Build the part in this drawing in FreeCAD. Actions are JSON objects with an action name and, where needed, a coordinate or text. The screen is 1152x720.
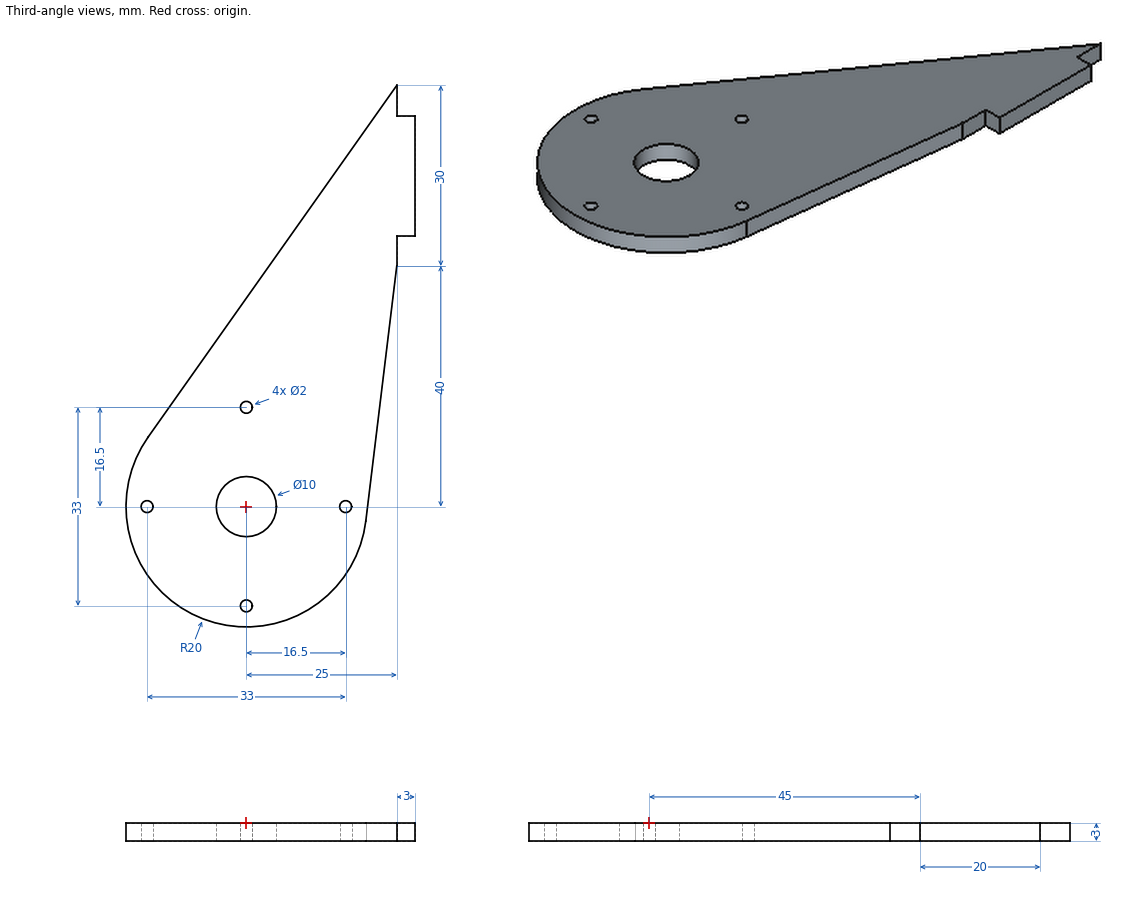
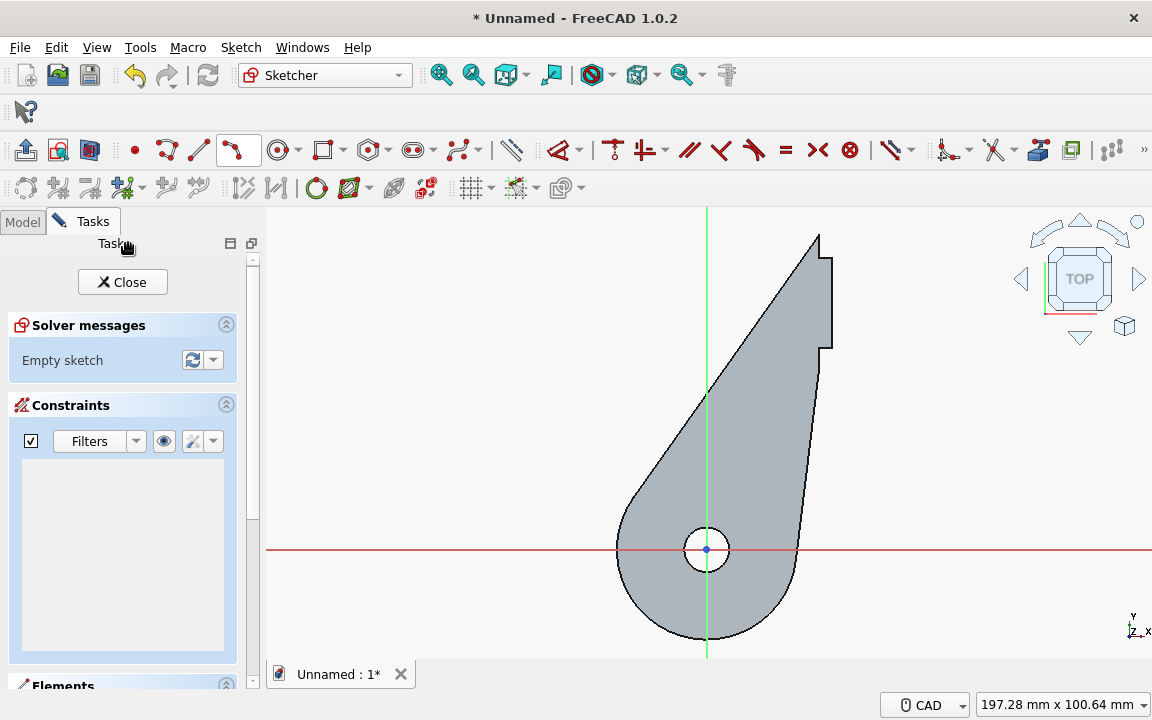
{"action": "scroll", "coordinate": [640, 433], "scroll_direction": "down", "scroll_amount": 5}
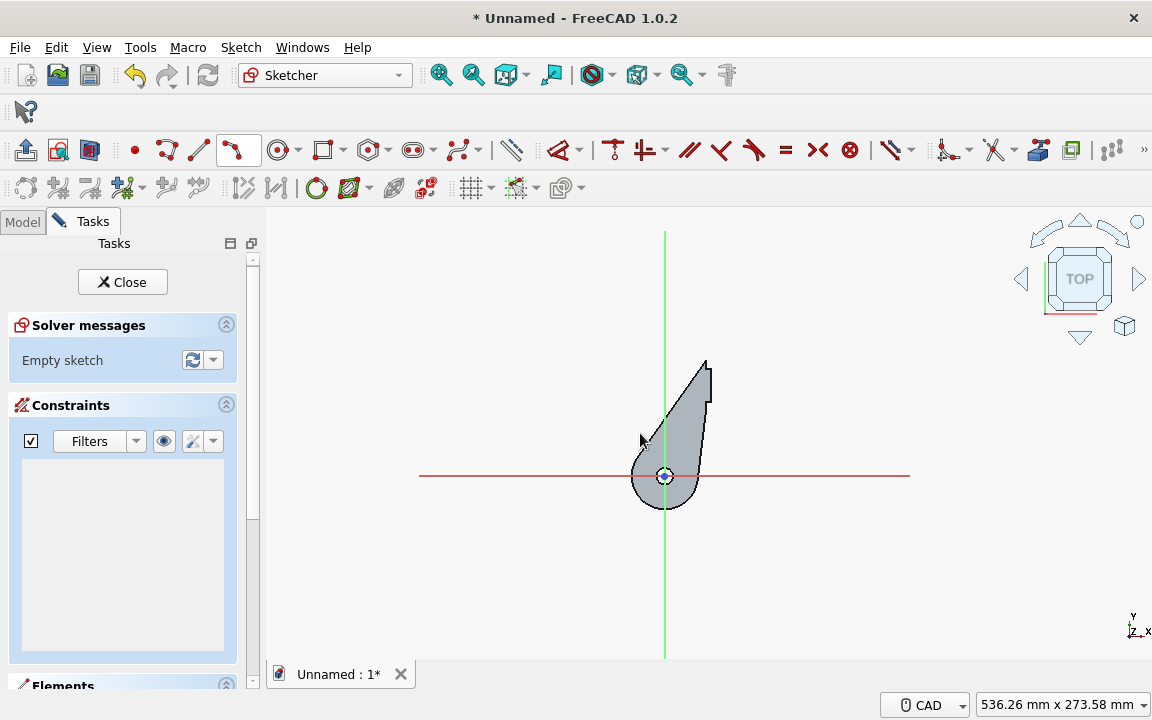
{"action": "scroll", "coordinate": [671, 487], "scroll_direction": "up", "scroll_amount": 8}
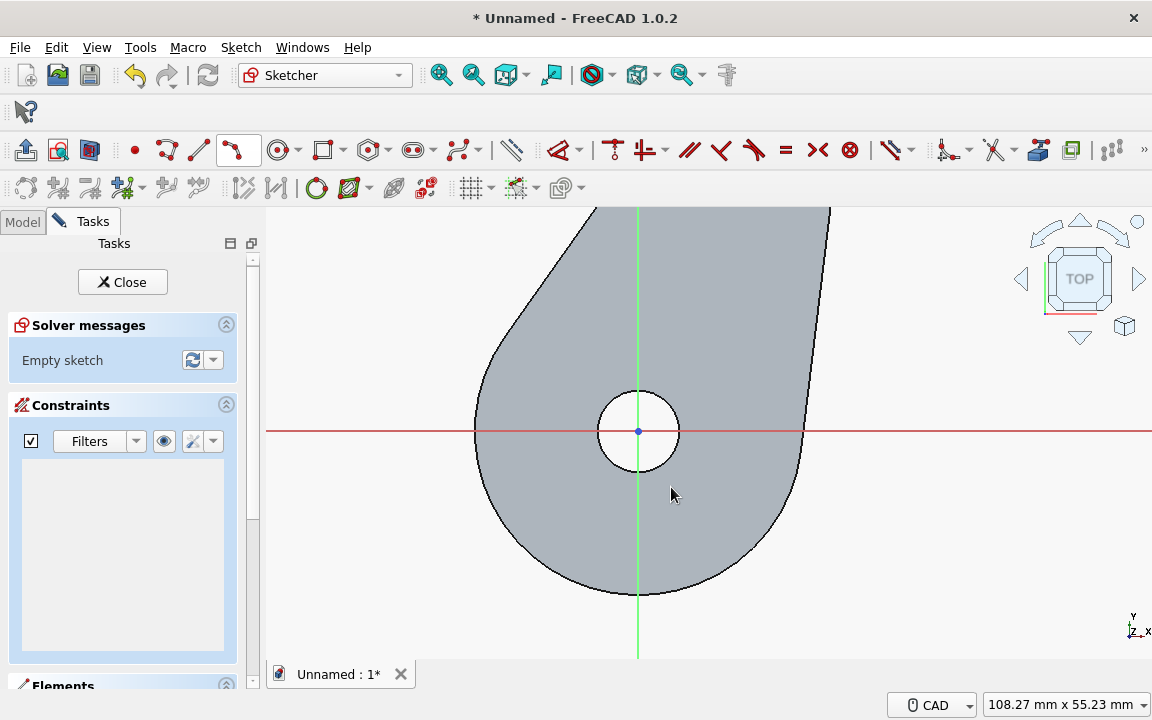
{"action": "left_click", "coordinate": [278, 150]}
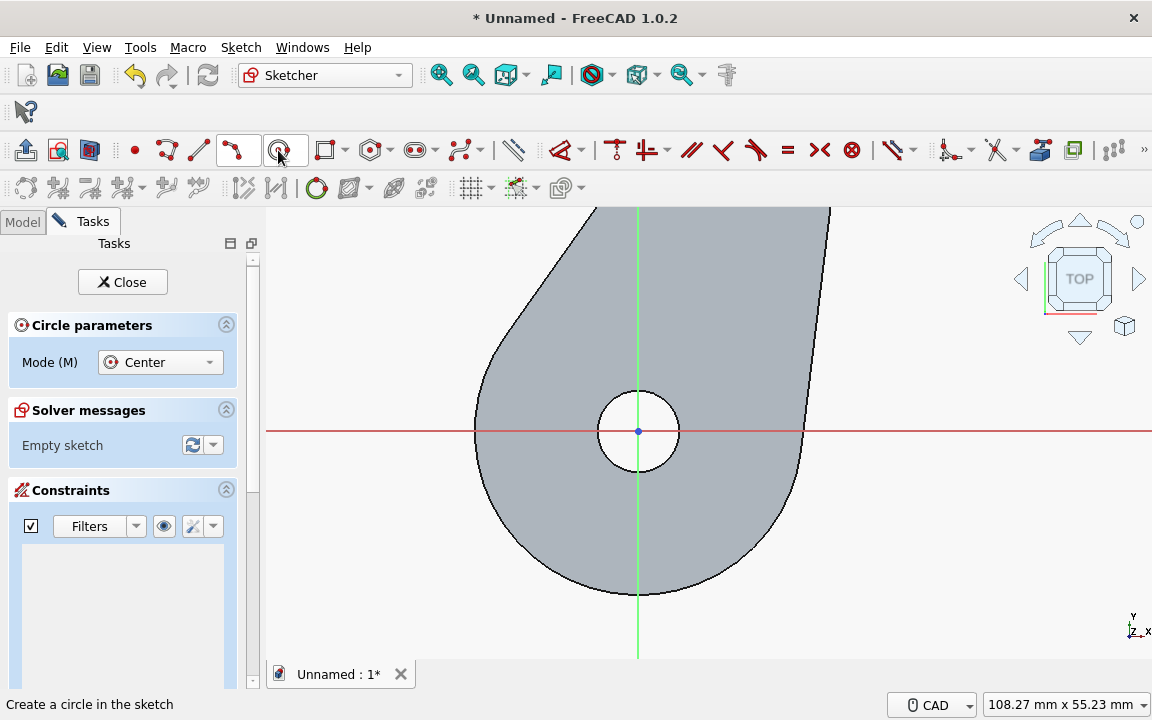
{"action": "scroll", "coordinate": [638, 296], "scroll_direction": "up", "scroll_amount": 6}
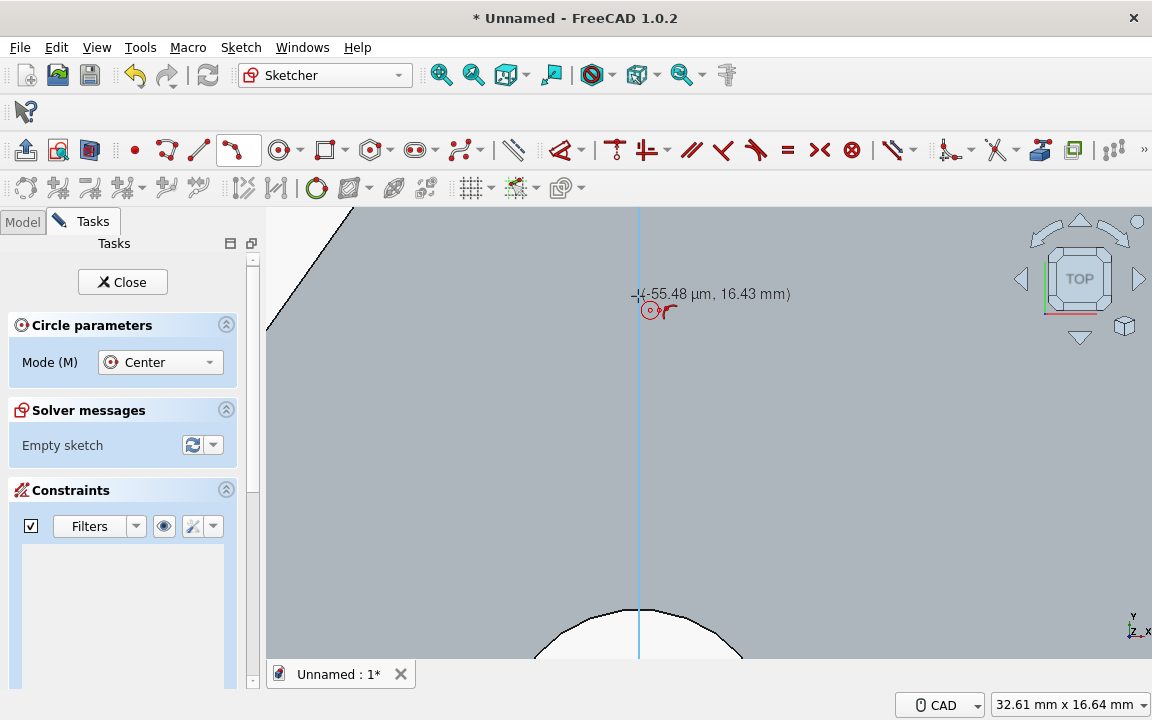
{"action": "left_click", "coordinate": [639, 297]}
{"action": "left_click", "coordinate": [658, 278]}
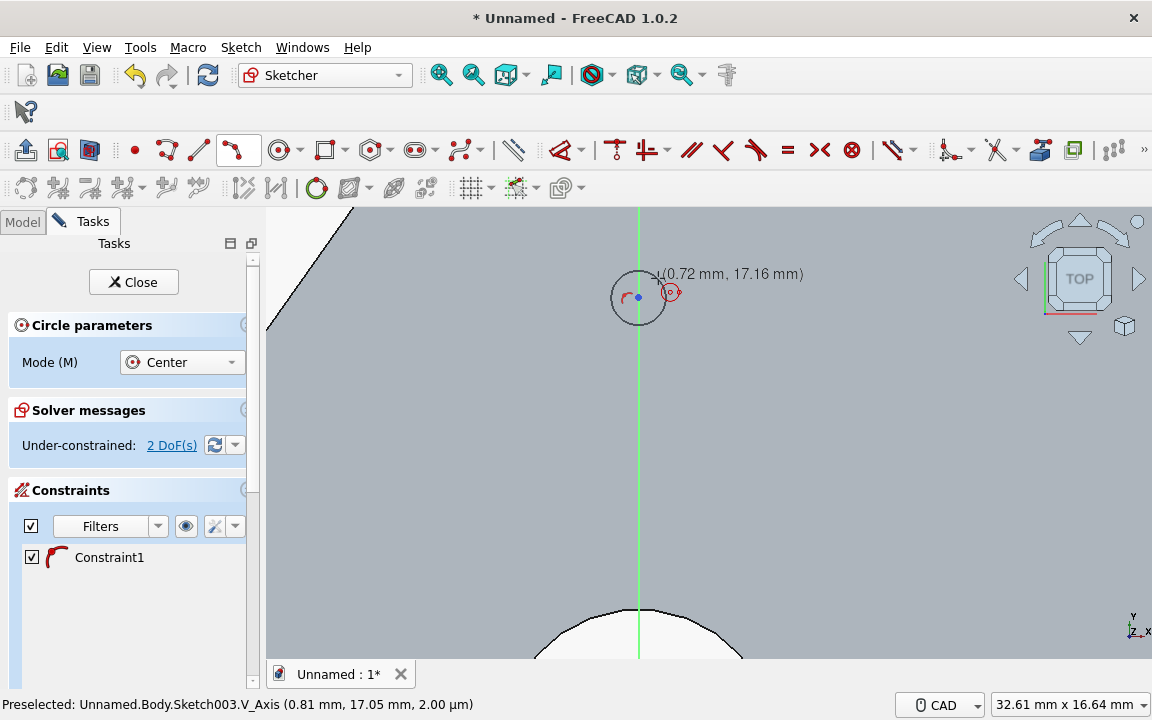
{"action": "scroll", "coordinate": [641, 298], "scroll_direction": "down", "scroll_amount": 6}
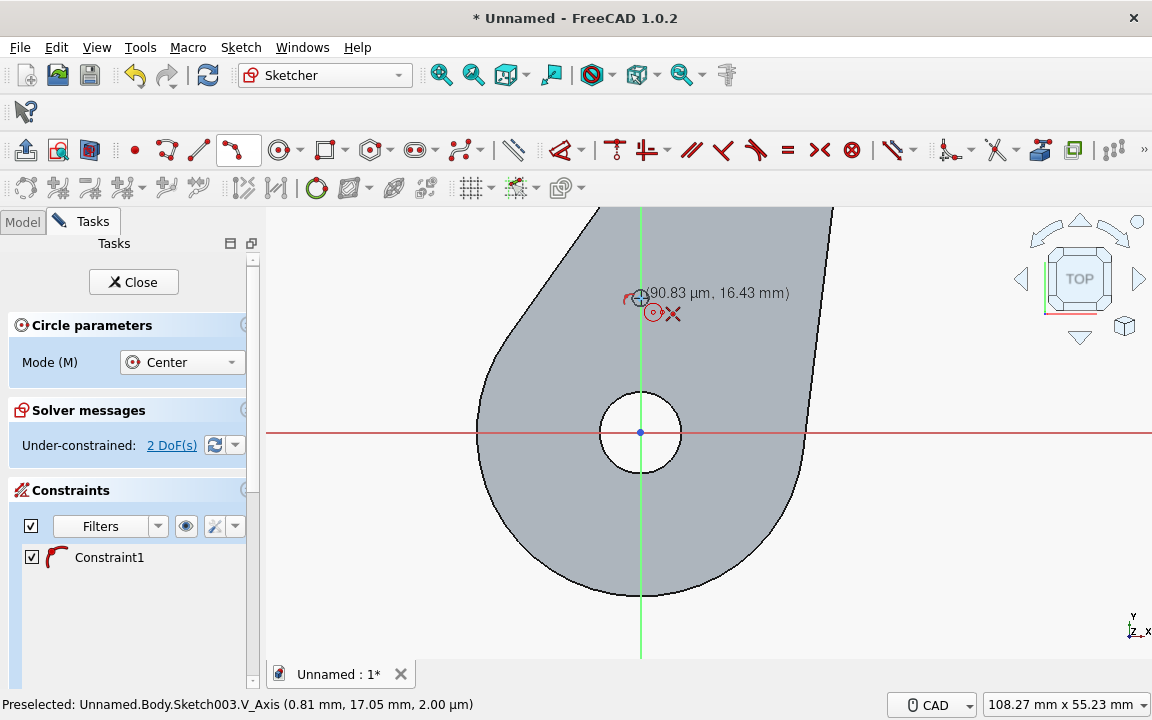
{"action": "scroll", "coordinate": [641, 568], "scroll_direction": "up", "scroll_amount": 6}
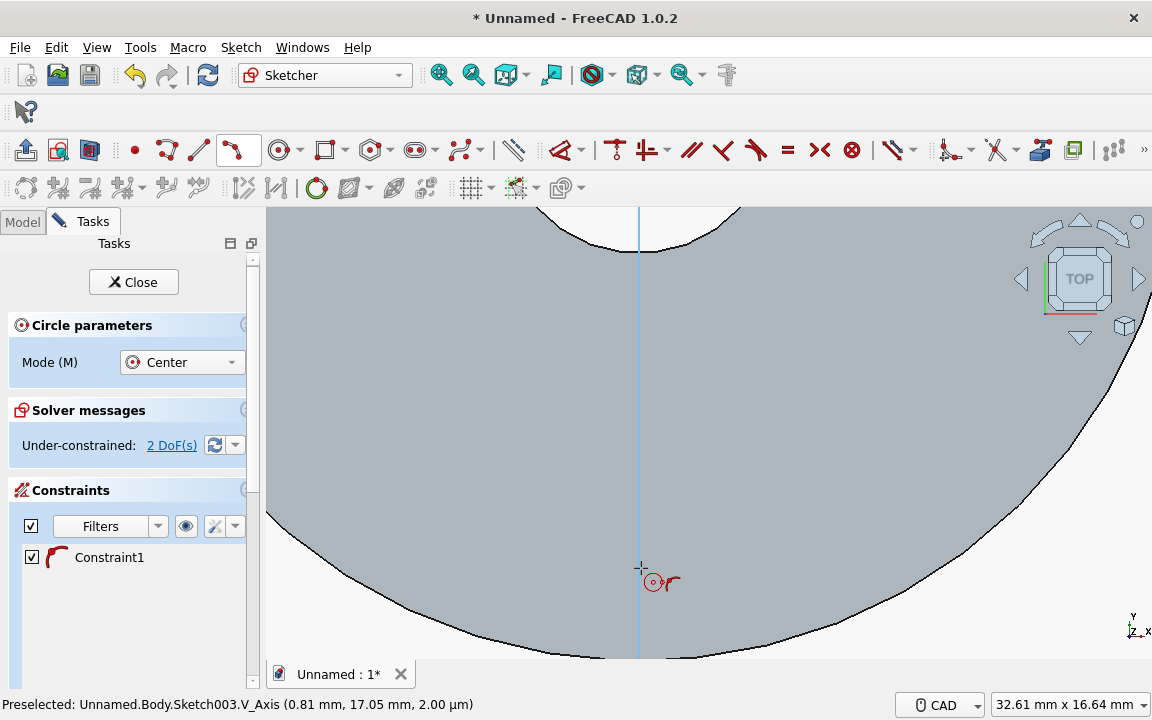
{"action": "left_click", "coordinate": [639, 566]}
{"action": "left_click", "coordinate": [658, 547]}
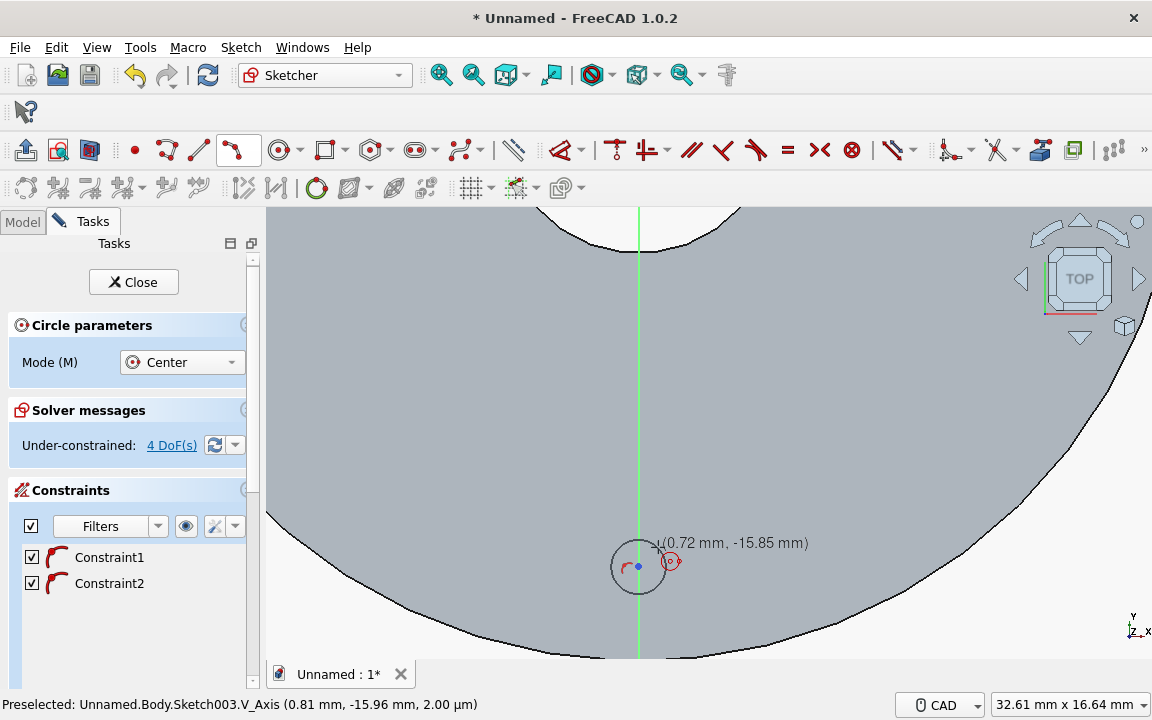
{"action": "scroll", "coordinate": [641, 569], "scroll_direction": "down", "scroll_amount": 6}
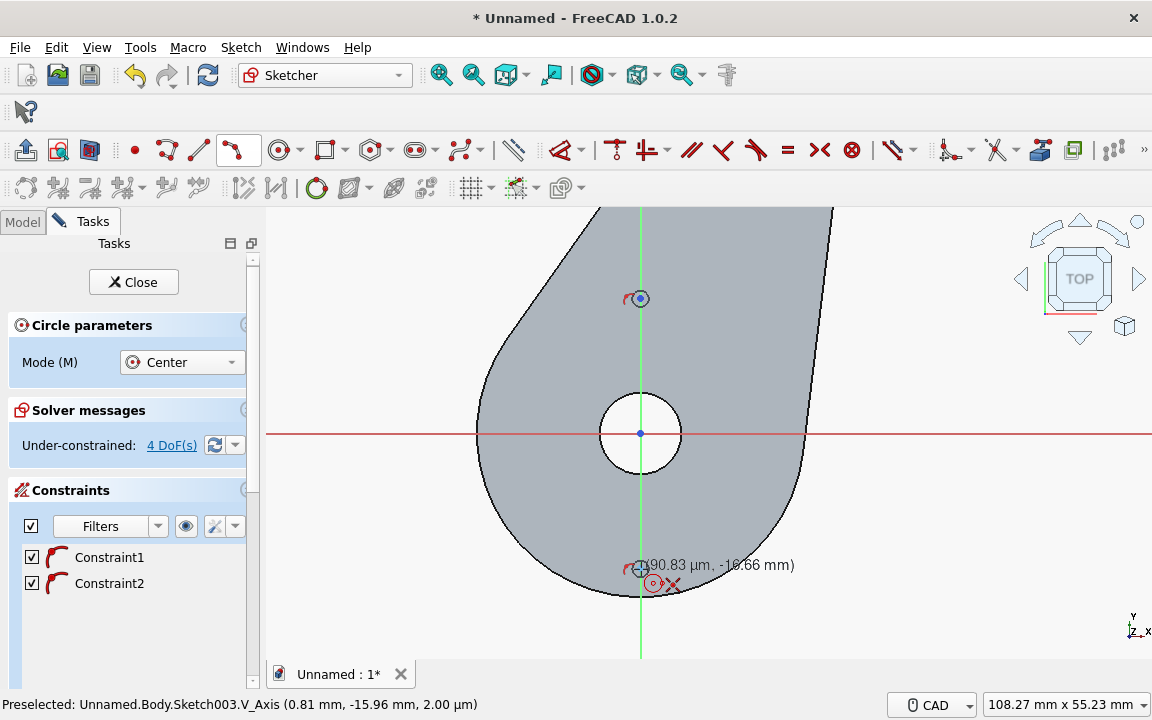
{"action": "scroll", "coordinate": [776, 434], "scroll_direction": "up", "scroll_amount": 6}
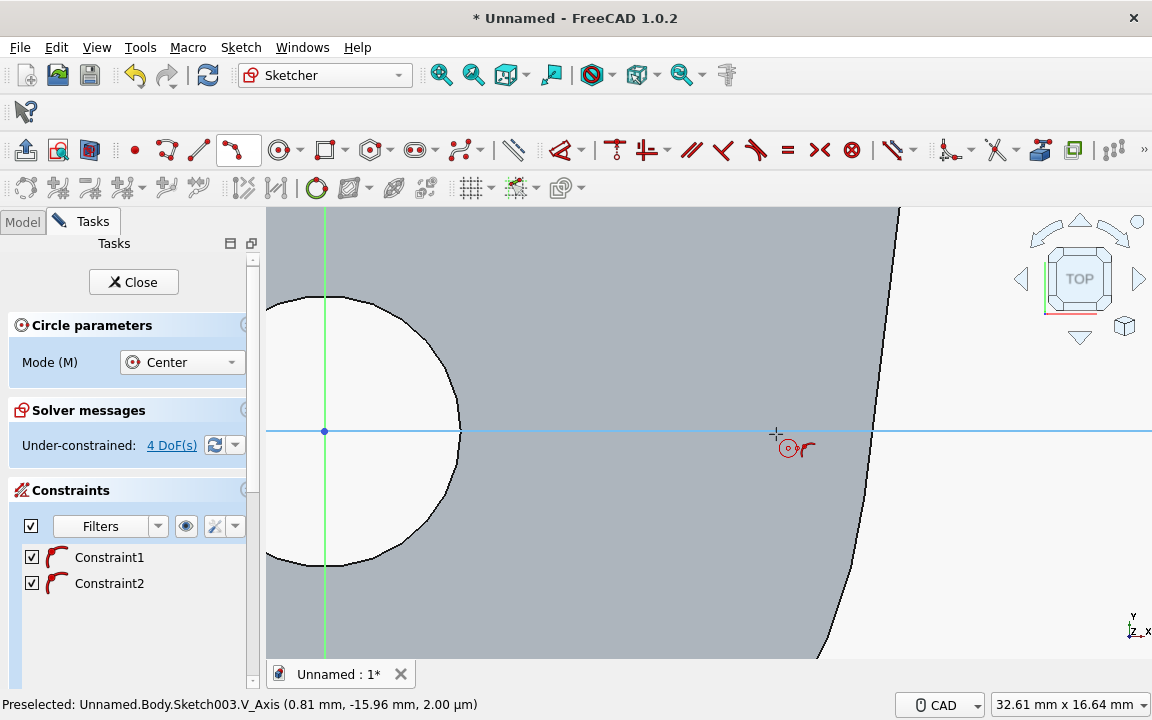
{"action": "left_click", "coordinate": [773, 431]}
{"action": "left_click", "coordinate": [792, 412]}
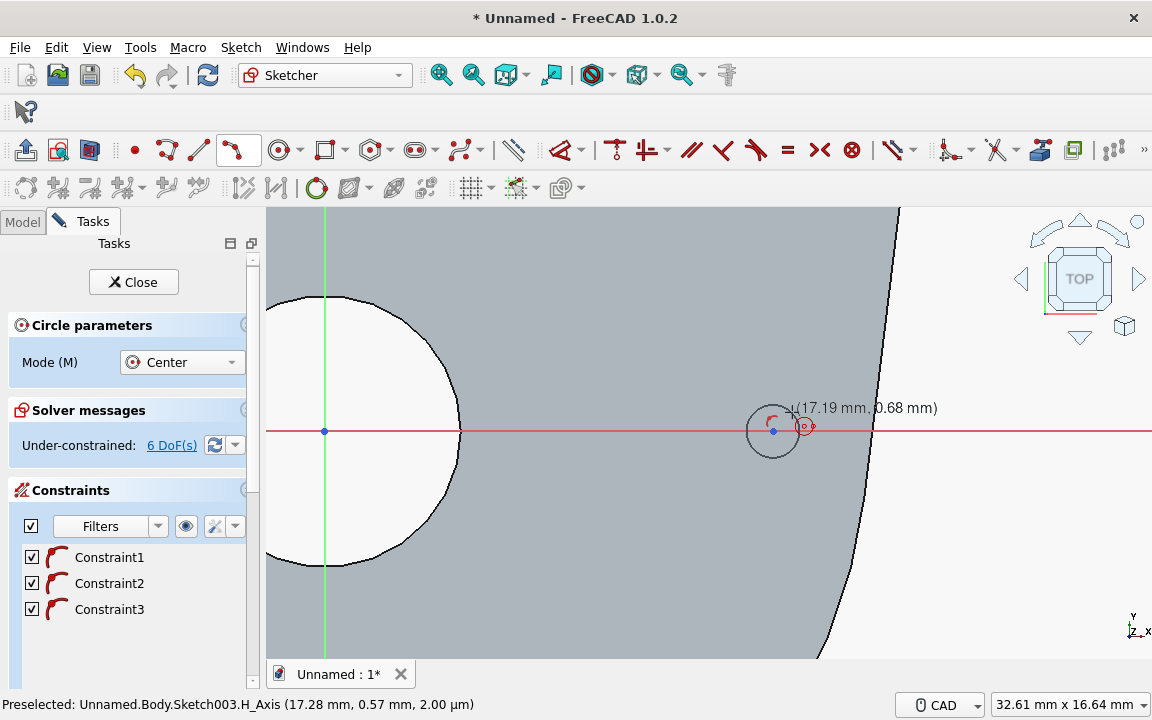
{"action": "scroll", "coordinate": [777, 434], "scroll_direction": "down", "scroll_amount": 6}